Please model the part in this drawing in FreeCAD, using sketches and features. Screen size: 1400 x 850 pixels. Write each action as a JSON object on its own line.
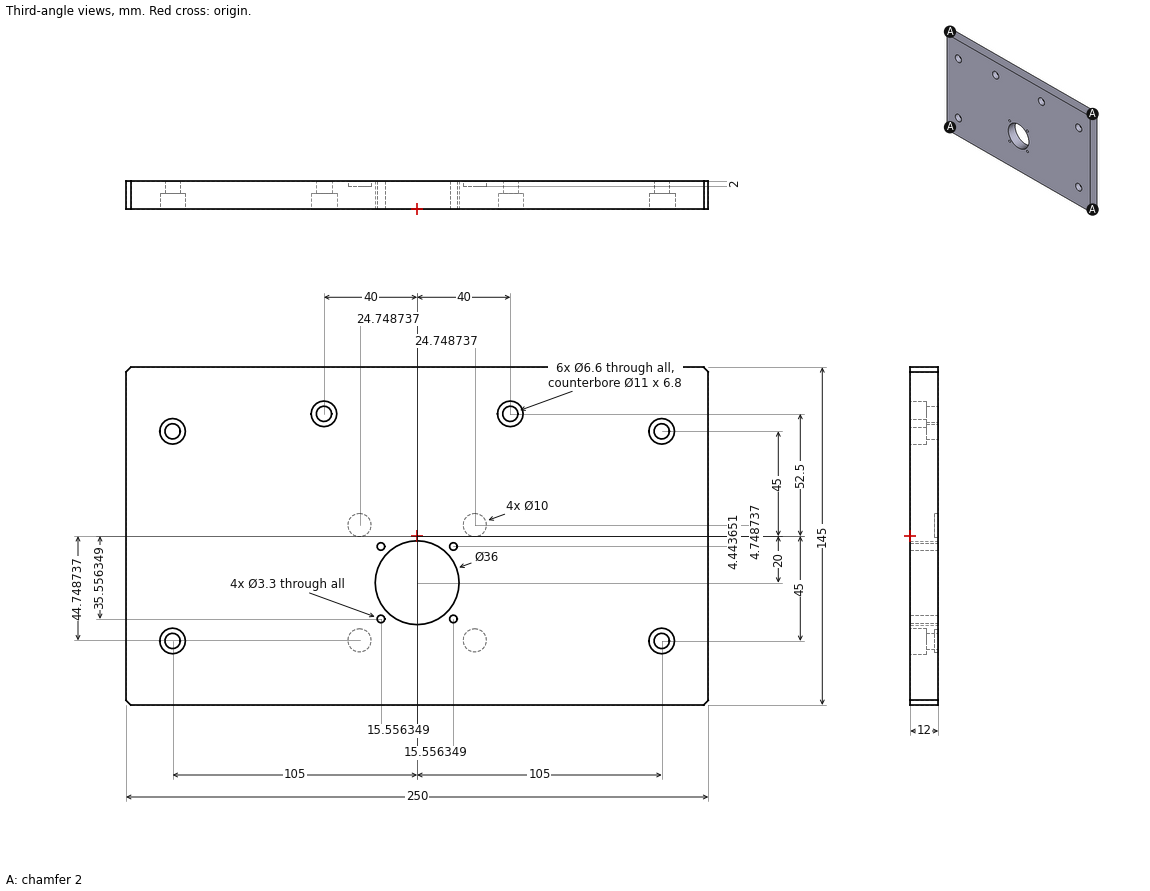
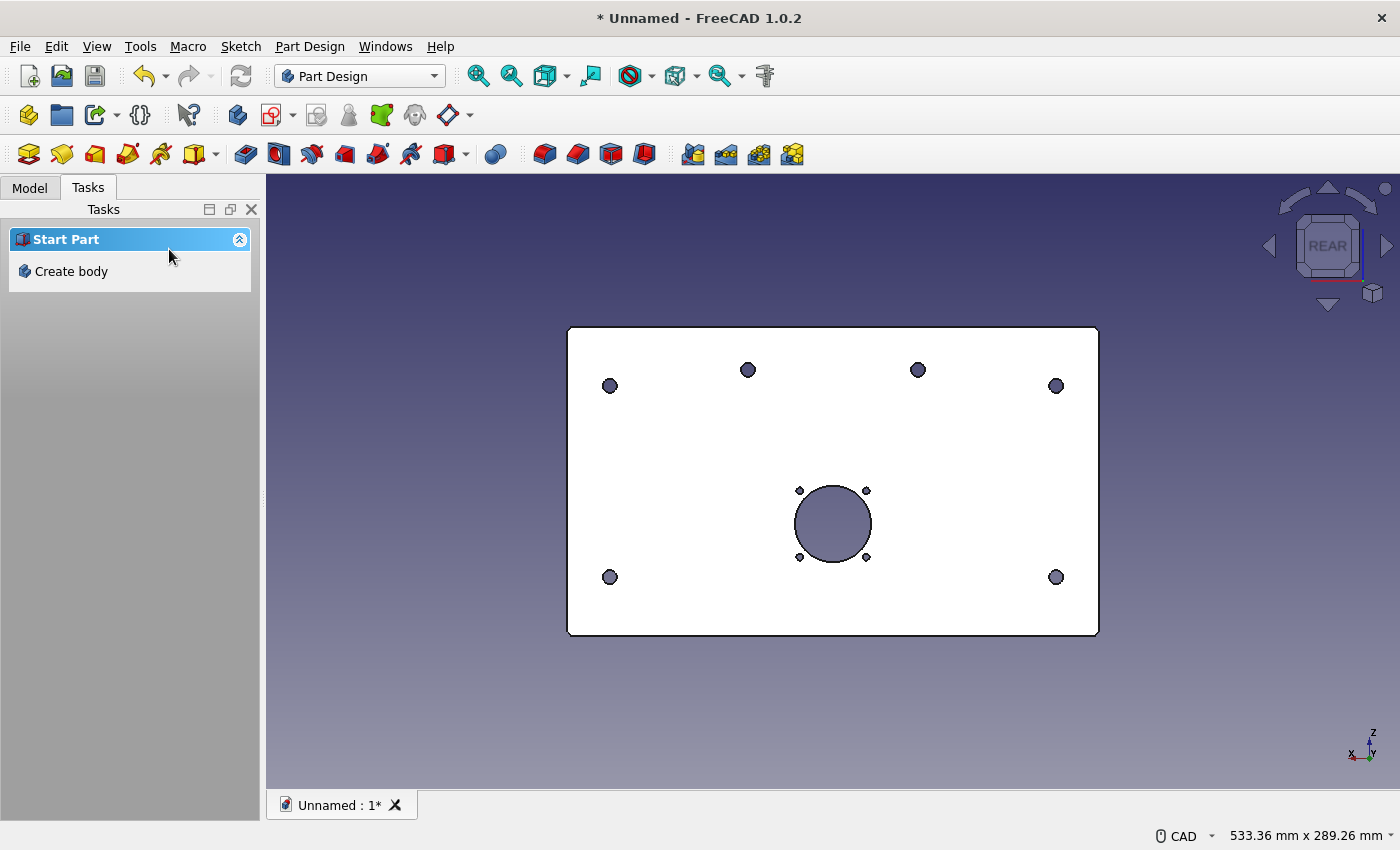
{"action": "left_click", "coordinate": [681, 480]}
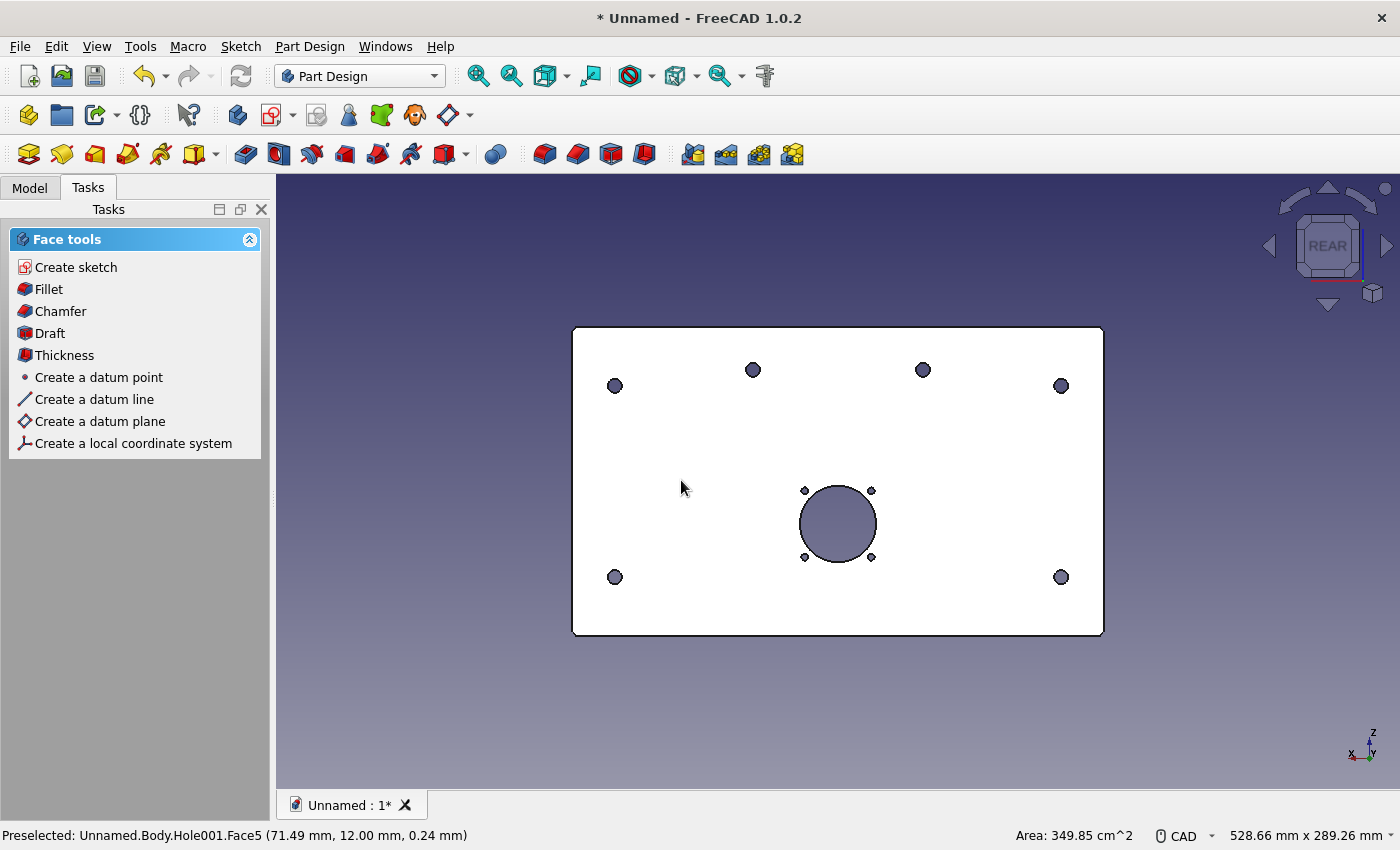
{"action": "left_click", "coordinate": [270, 116]}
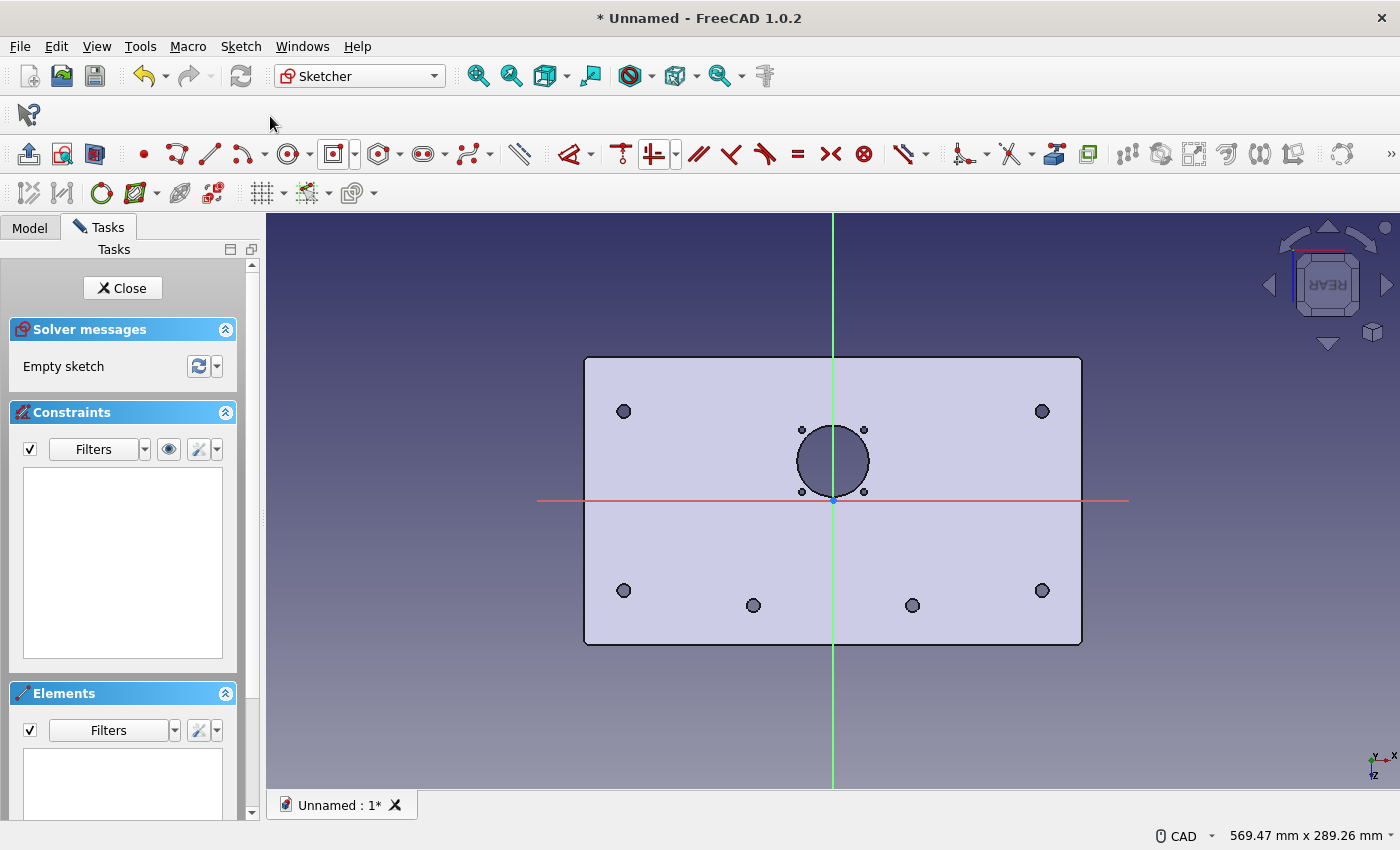
{"action": "scroll", "coordinate": [863, 444], "scroll_direction": "up", "scroll_amount": 6}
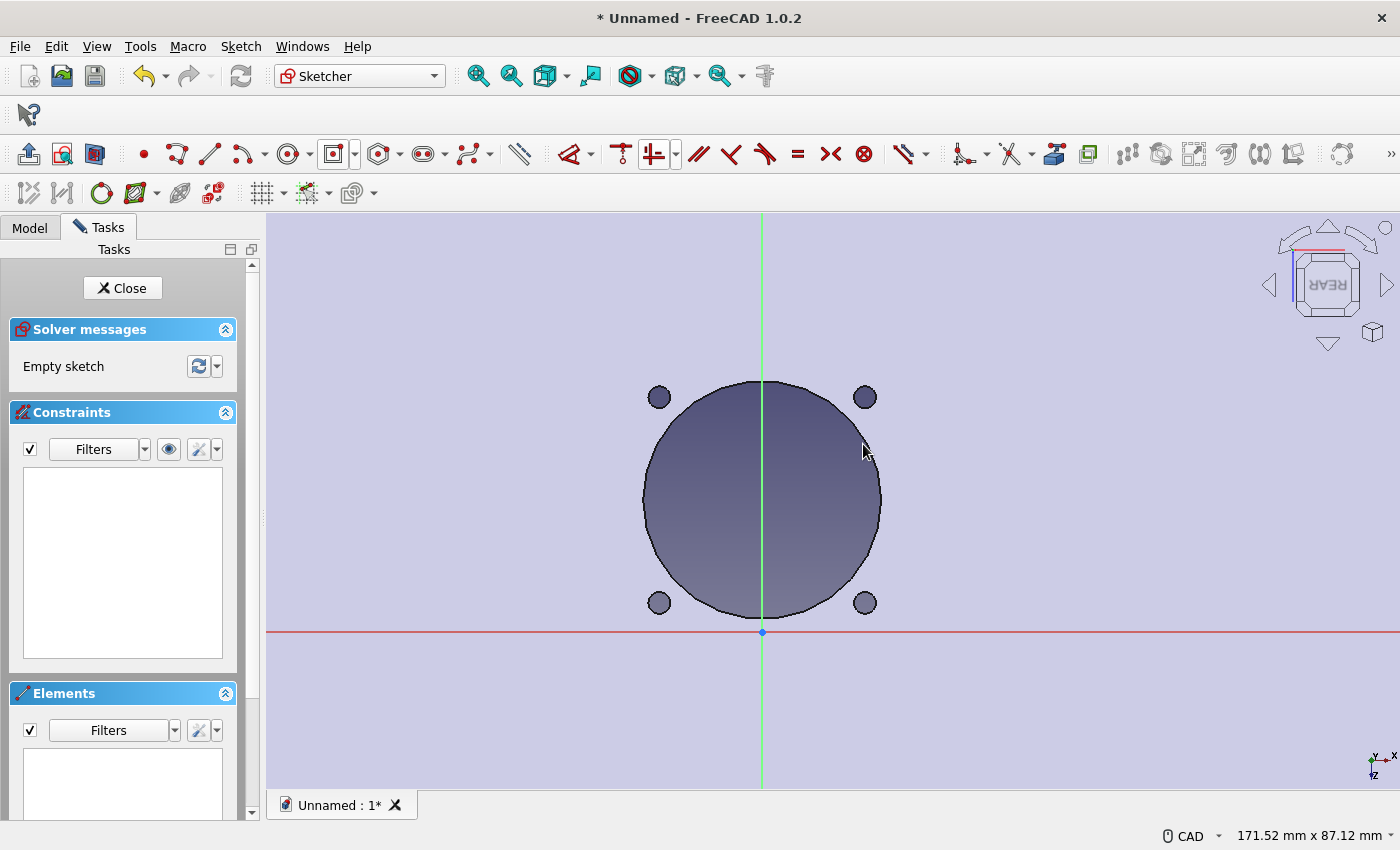
{"action": "key", "text": "g c"}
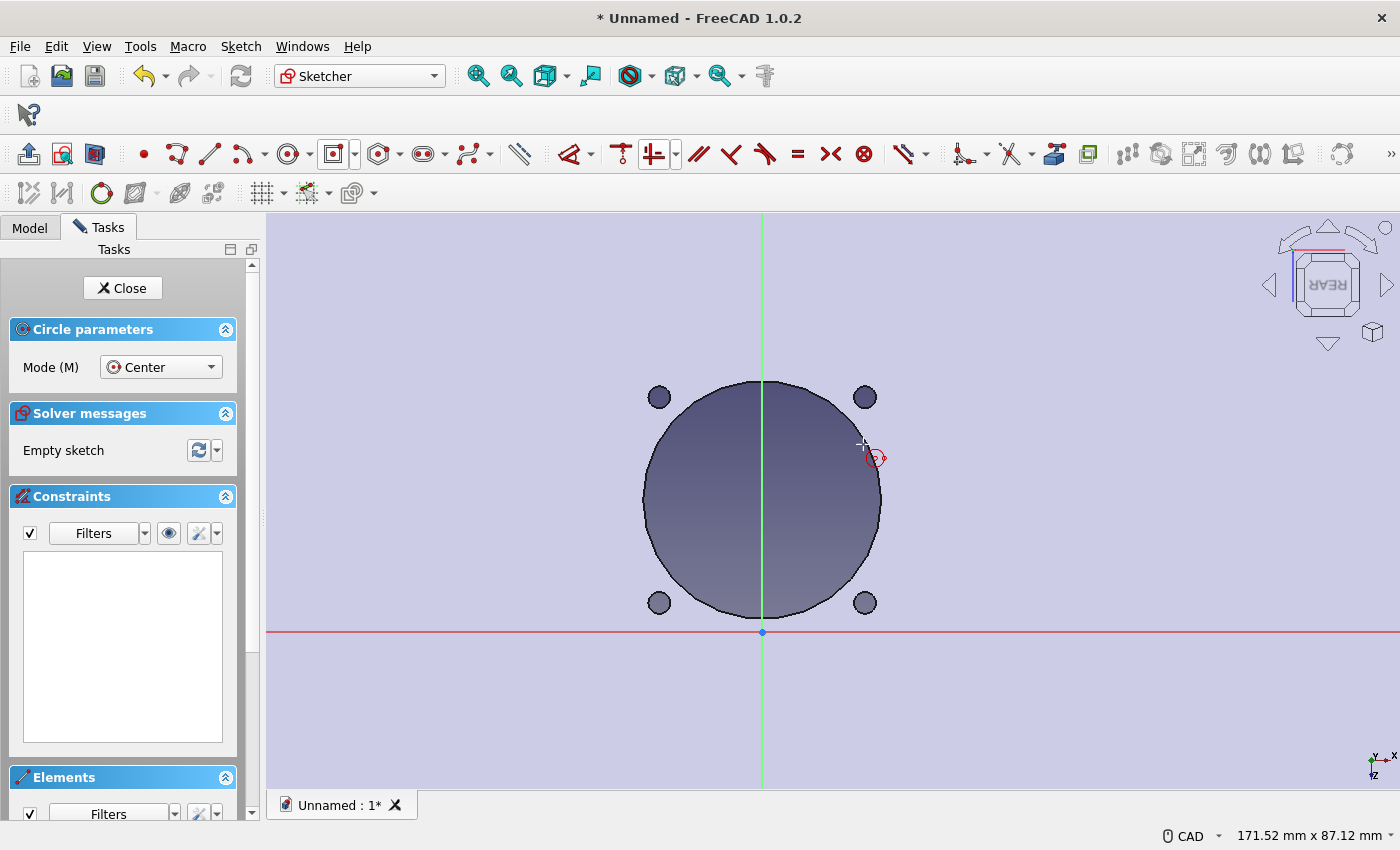
{"action": "left_click", "coordinate": [926, 664]}
{"action": "mouse_move", "coordinate": [949, 687]}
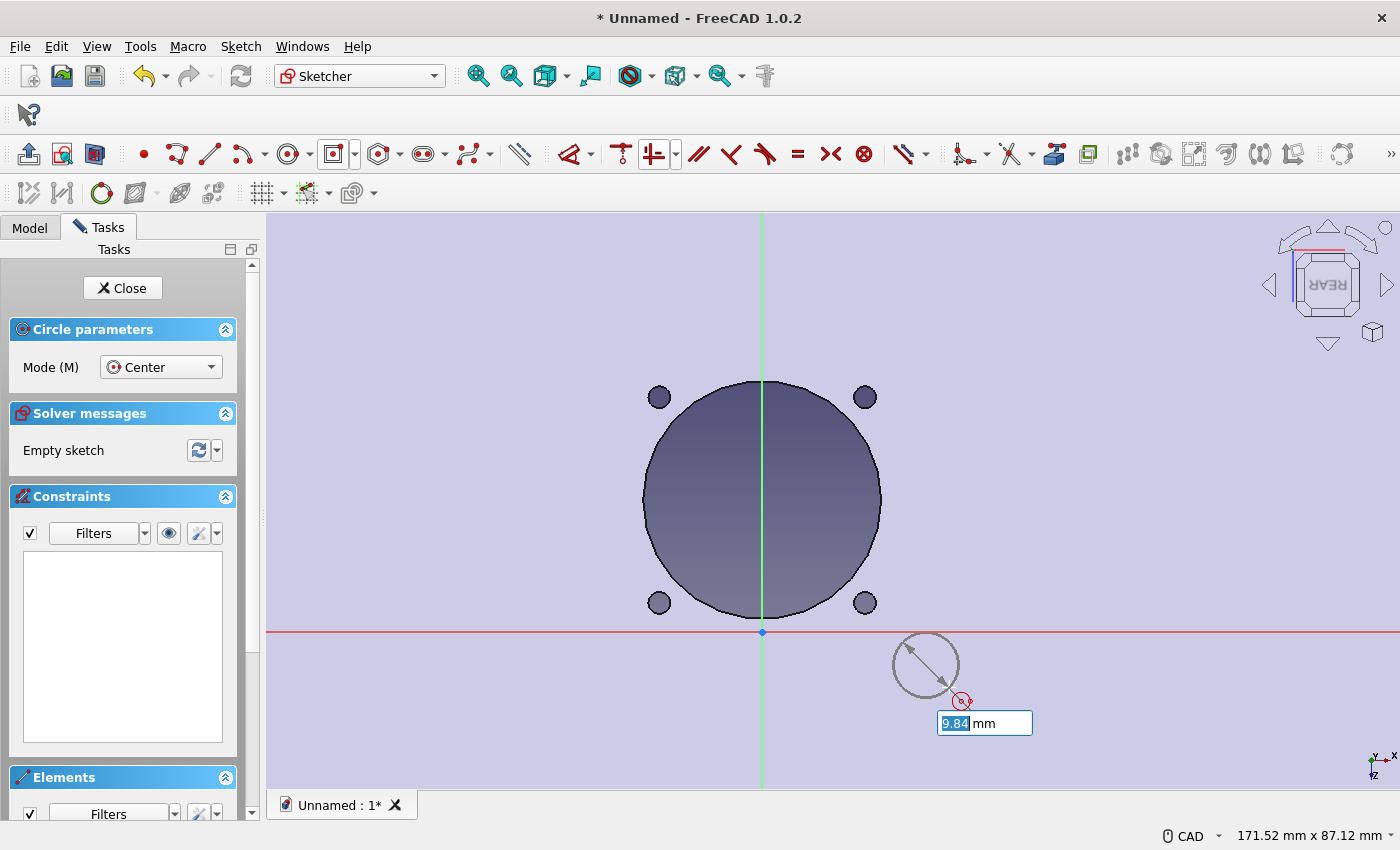
{"action": "type", "text": "10"}
{"action": "key", "text": "Return"}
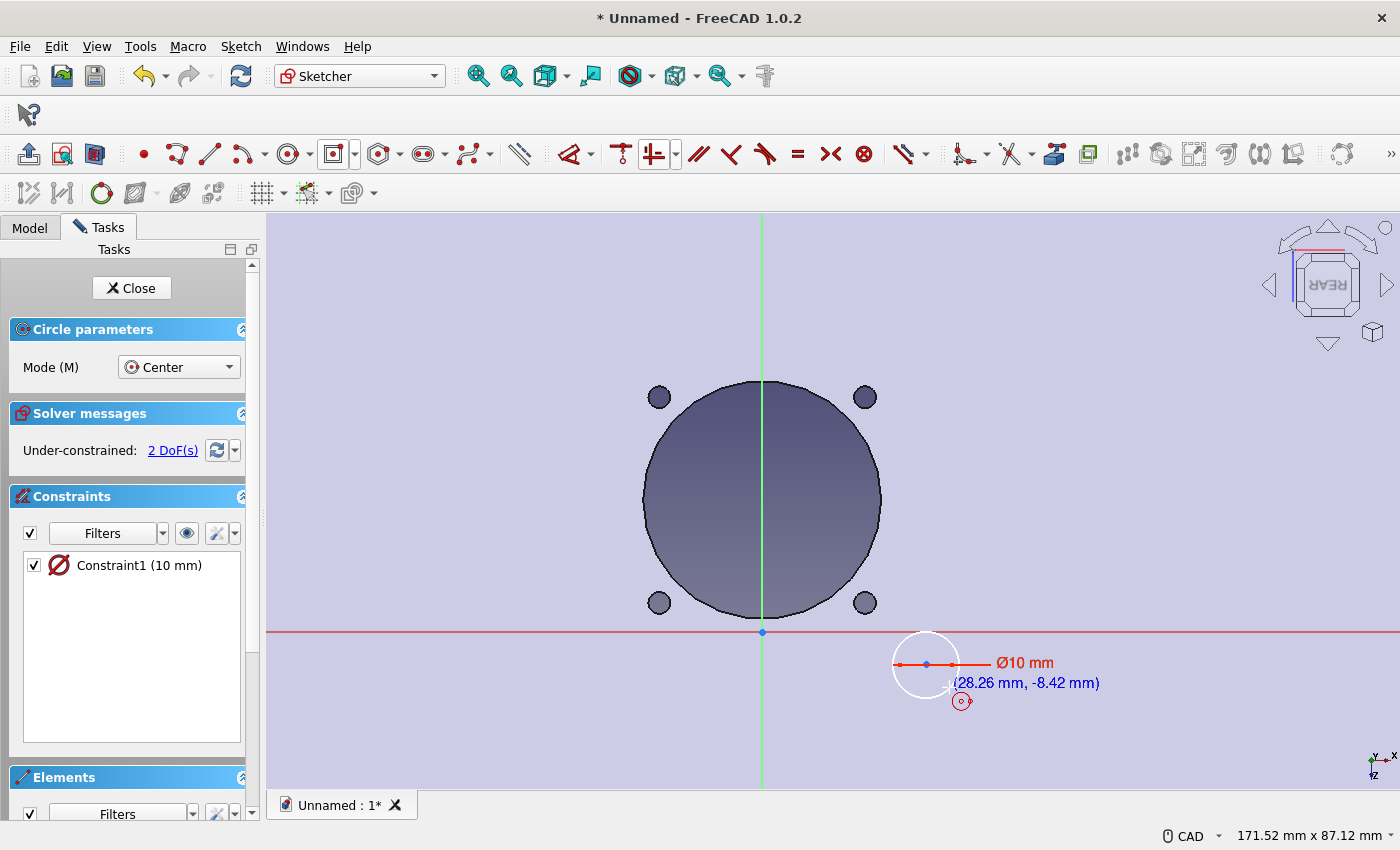
{"action": "left_click", "coordinate": [599, 664]}
{"action": "mouse_move", "coordinate": [622, 687]}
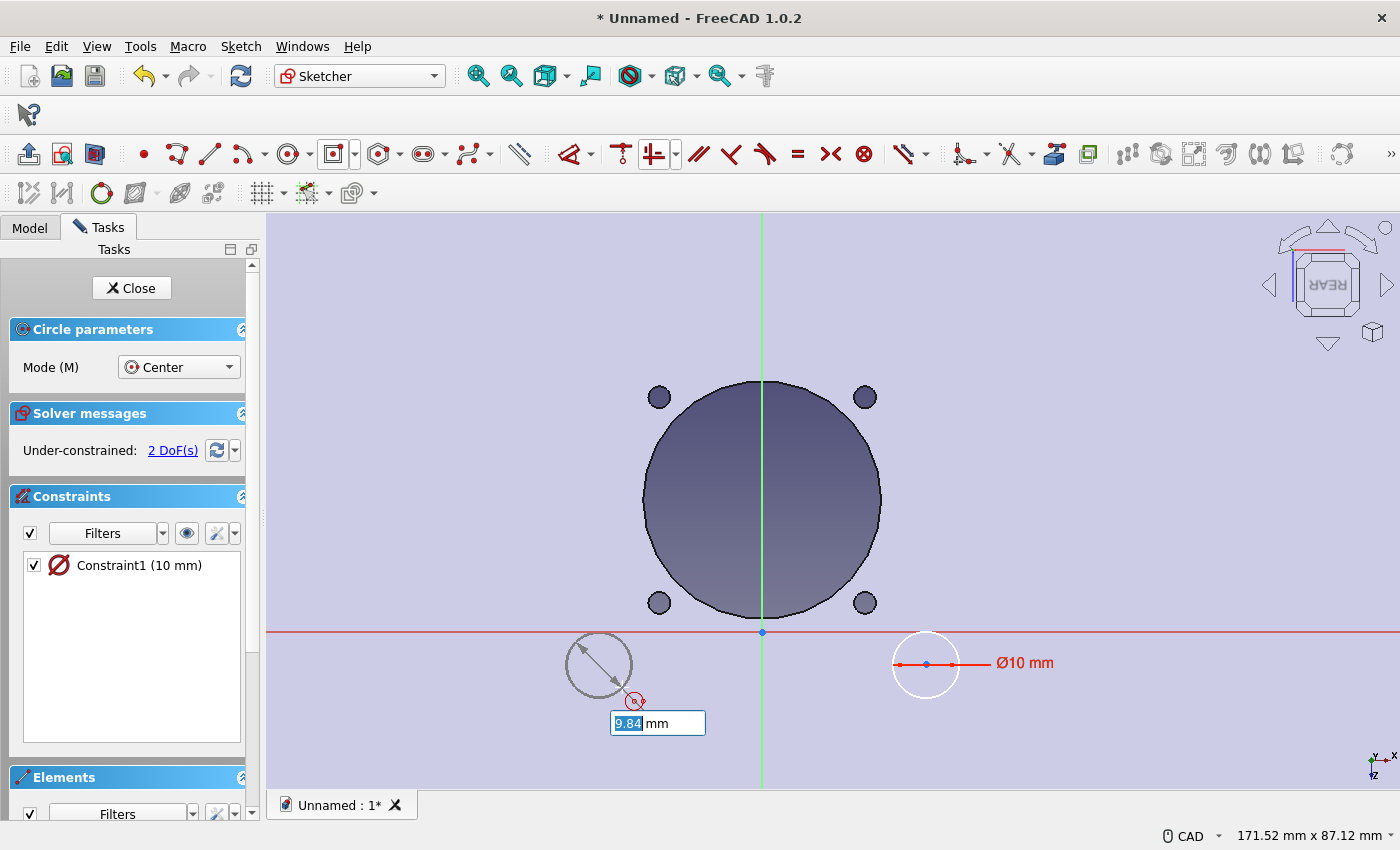
{"action": "type", "text": "10"}
{"action": "key", "text": "Return"}